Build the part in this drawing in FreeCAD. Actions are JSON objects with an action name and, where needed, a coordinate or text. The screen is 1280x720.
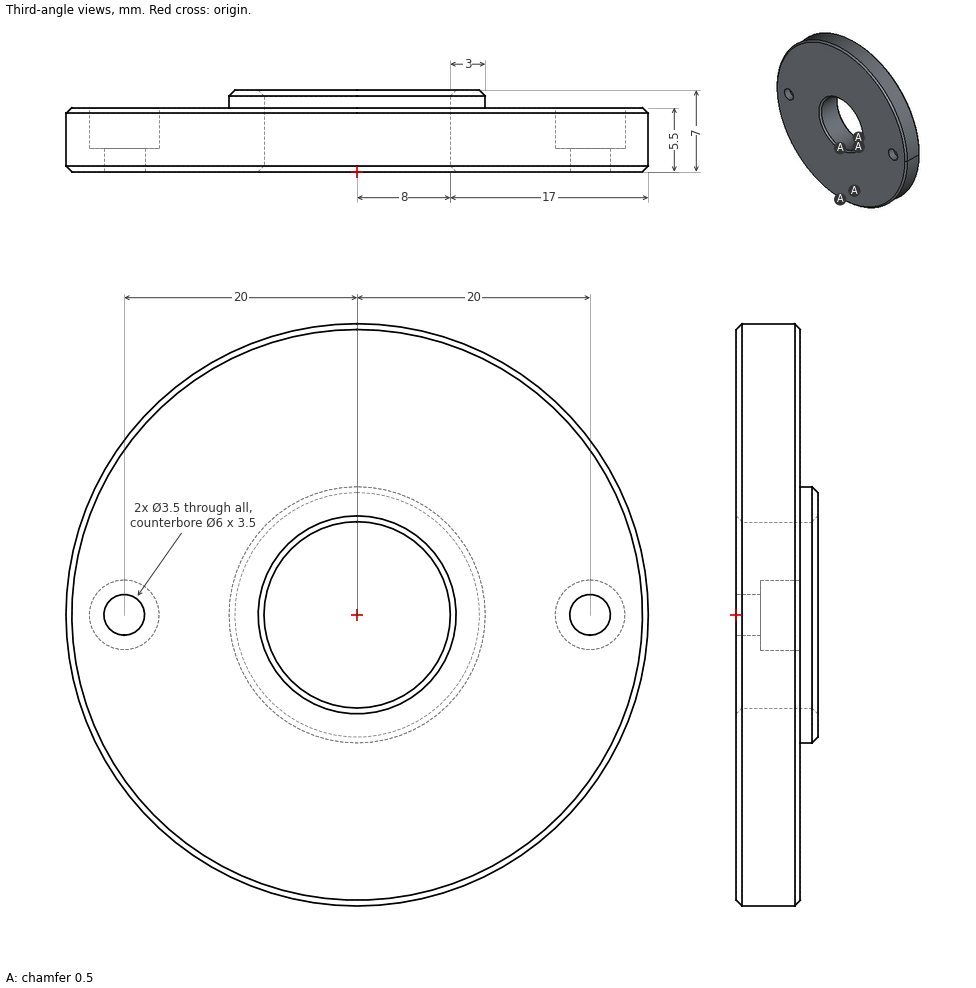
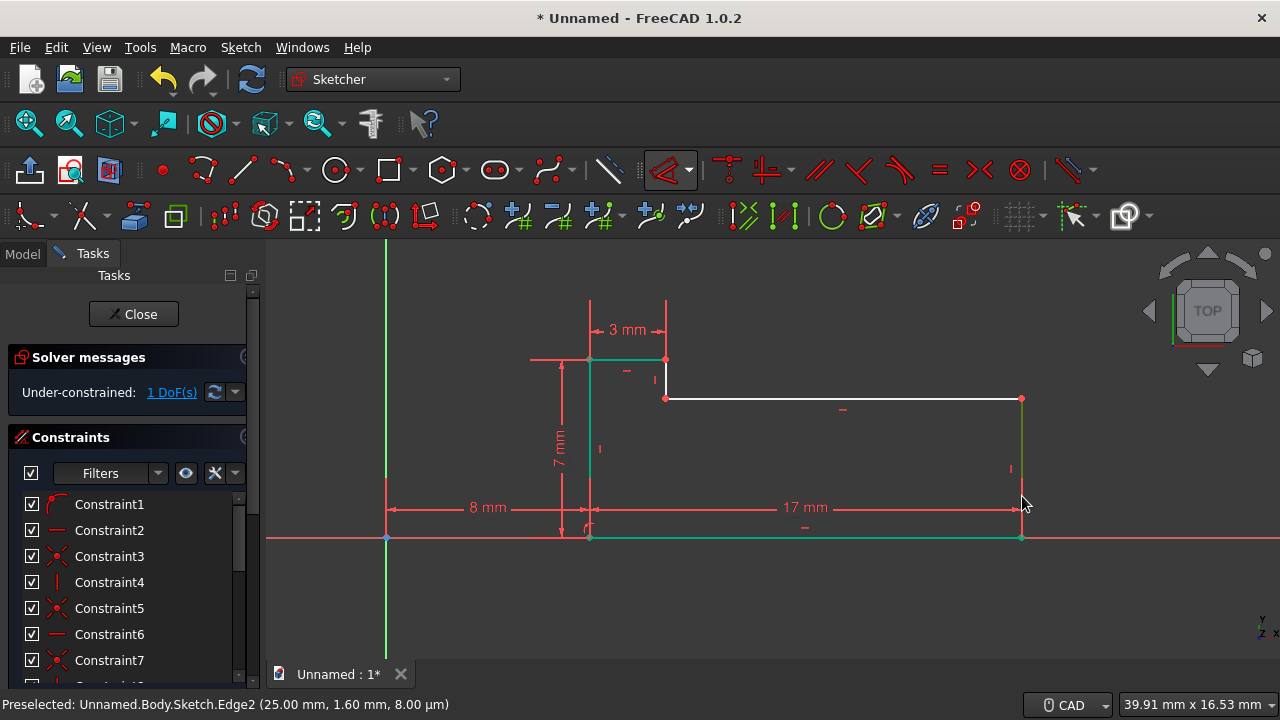
{"action": "left_click", "coordinate": [692, 170]}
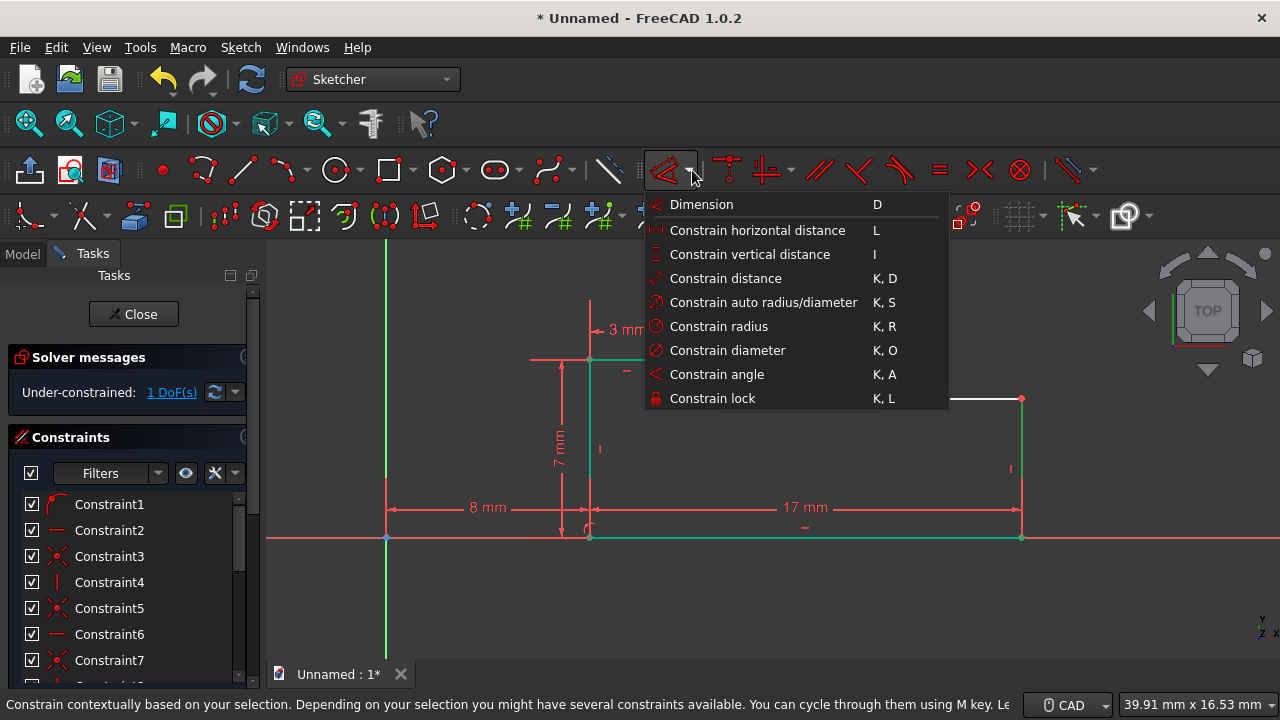
{"action": "left_click", "coordinate": [797, 254]}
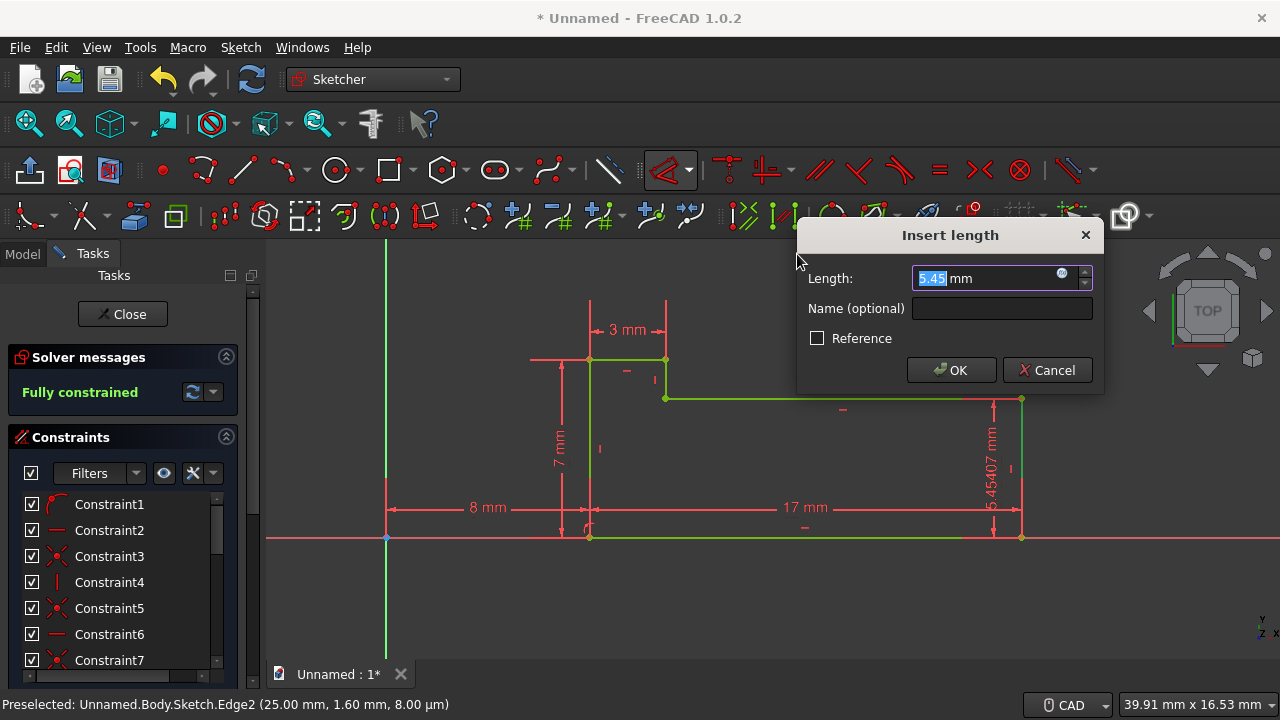
{"action": "type", "text": "5.5"}
{"action": "key", "text": "Return"}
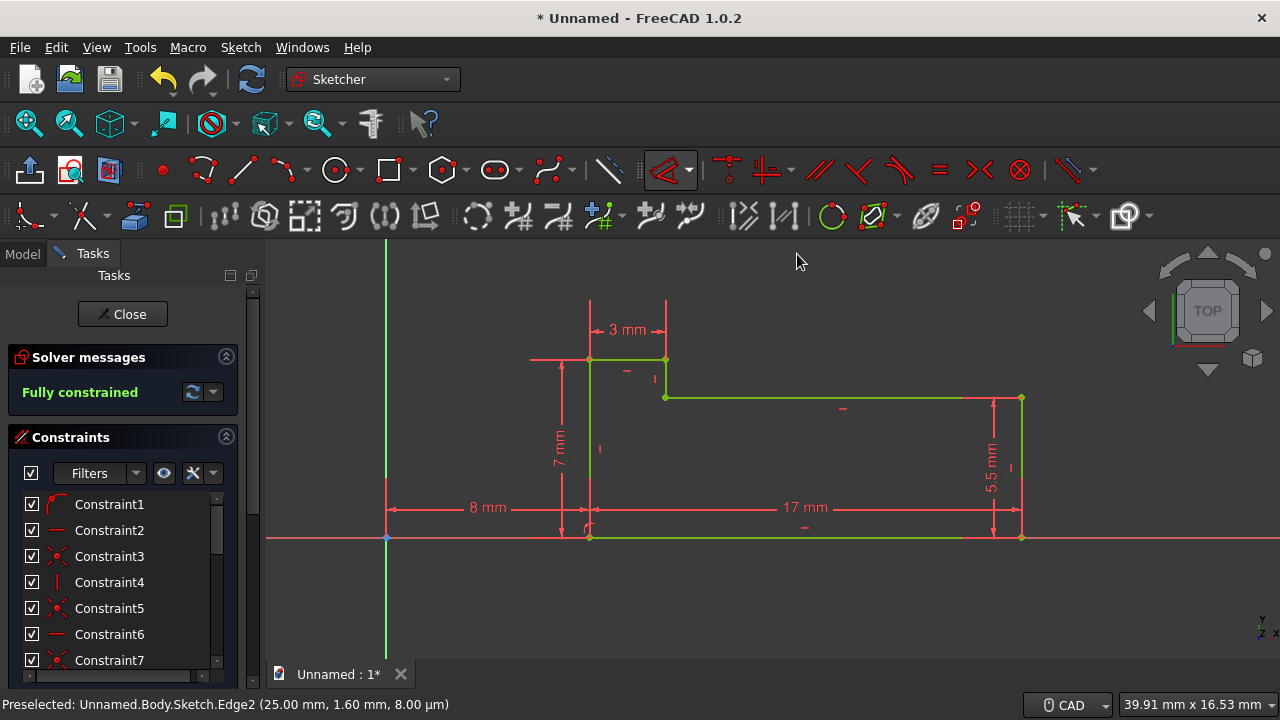
{"action": "left_click", "coordinate": [123, 314]}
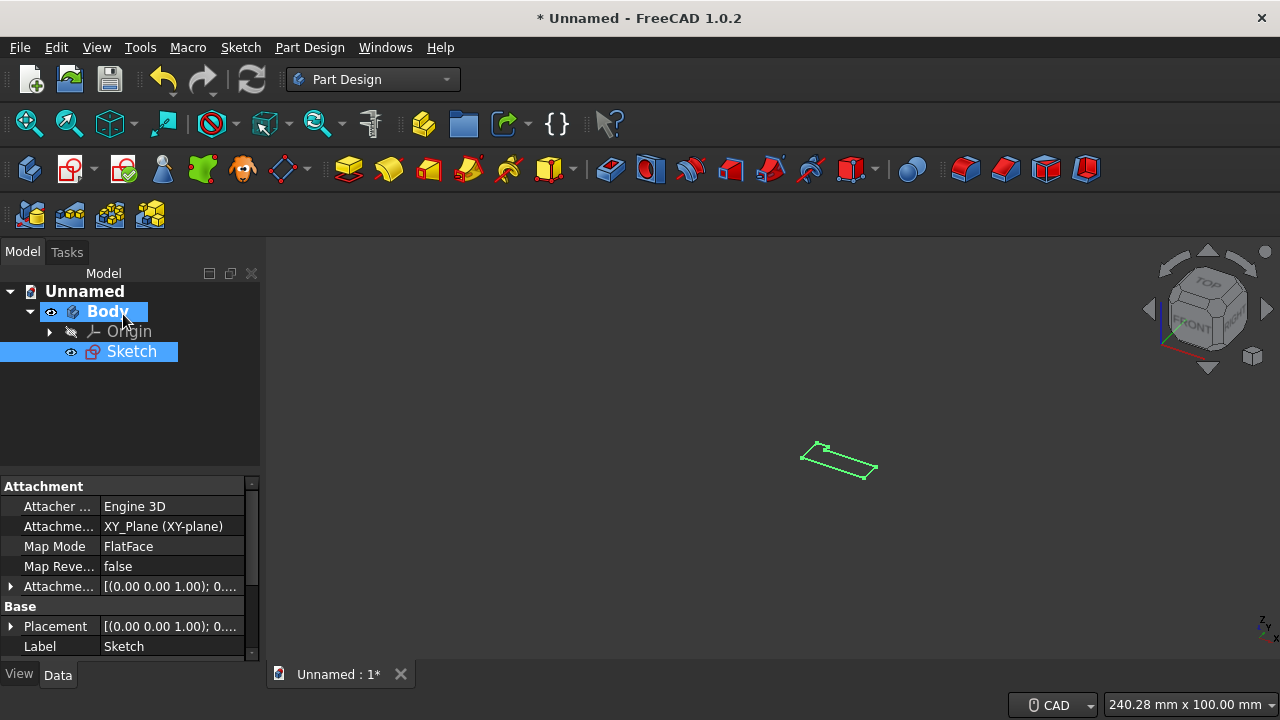
{"action": "left_click", "coordinate": [390, 170]}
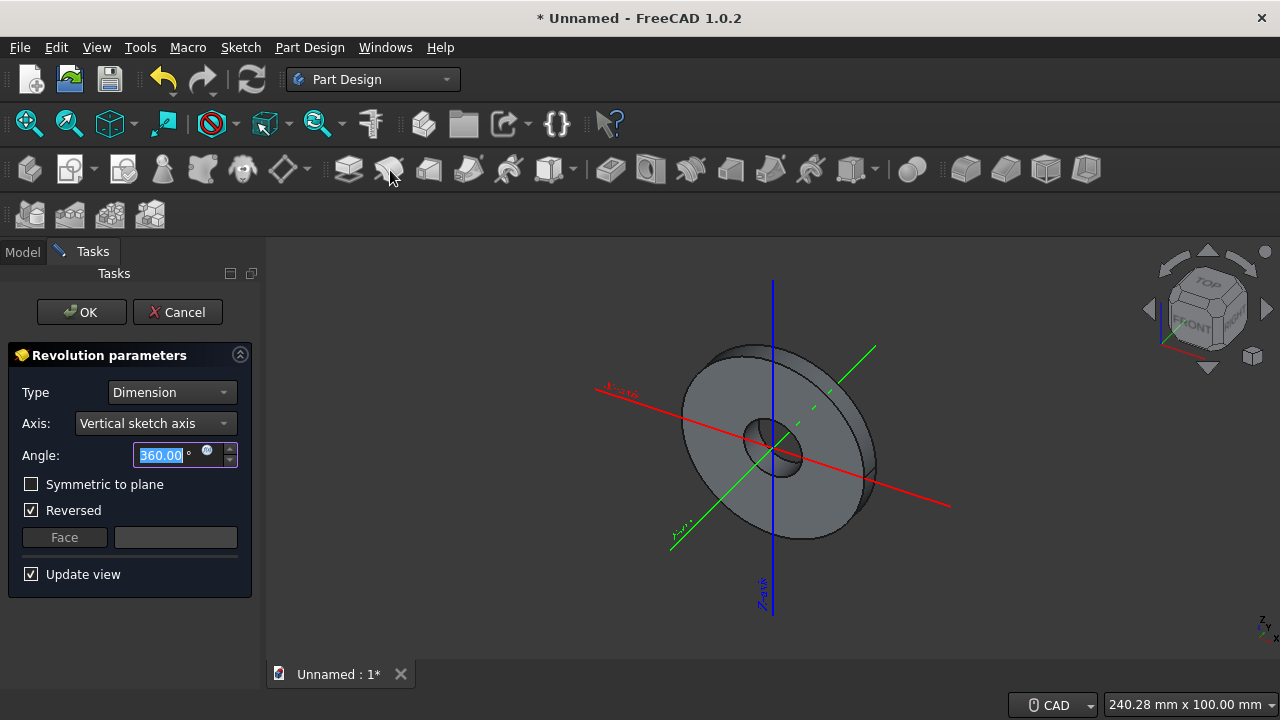
{"action": "left_click", "coordinate": [82, 312]}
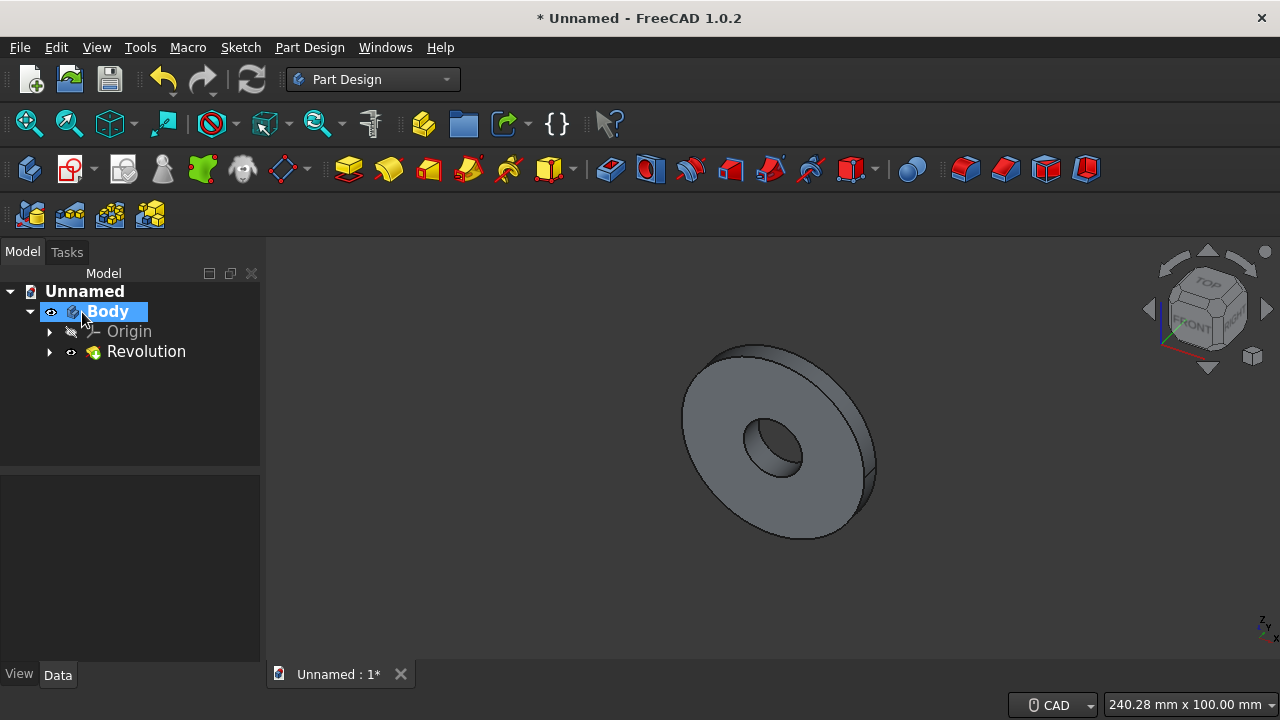
{"action": "key", "text": "4"}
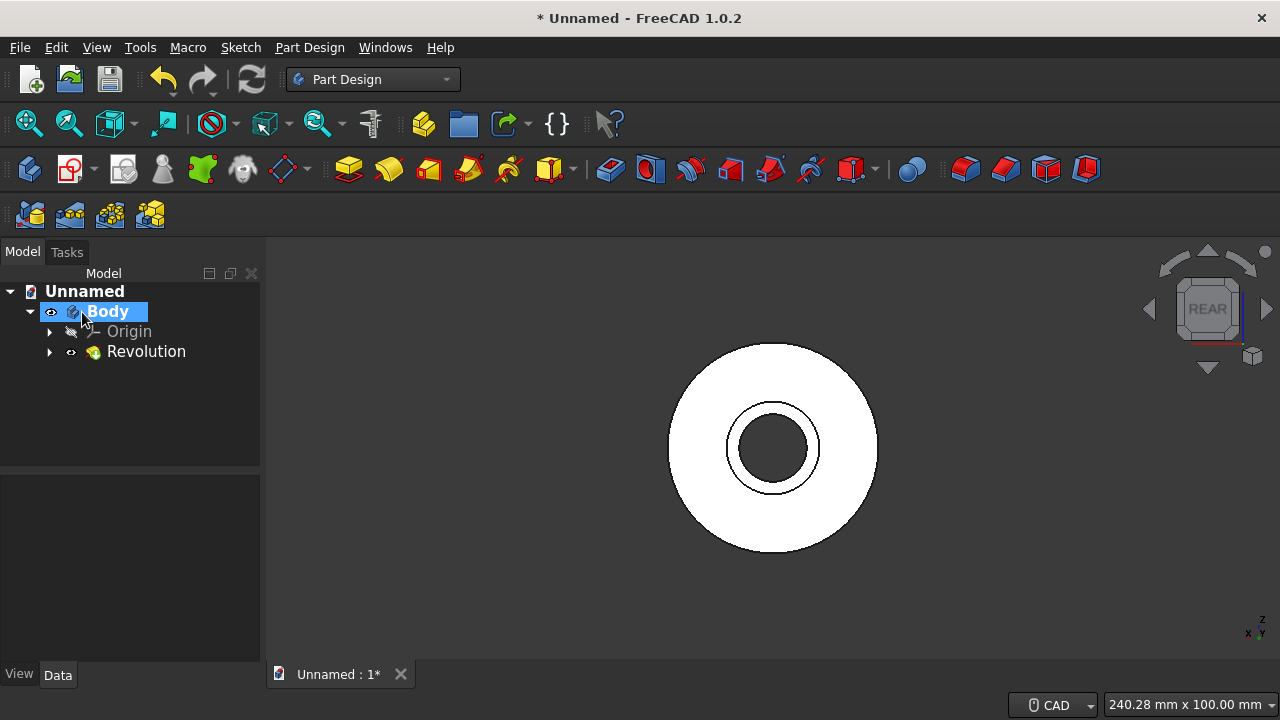
{"action": "left_click", "coordinate": [713, 417]}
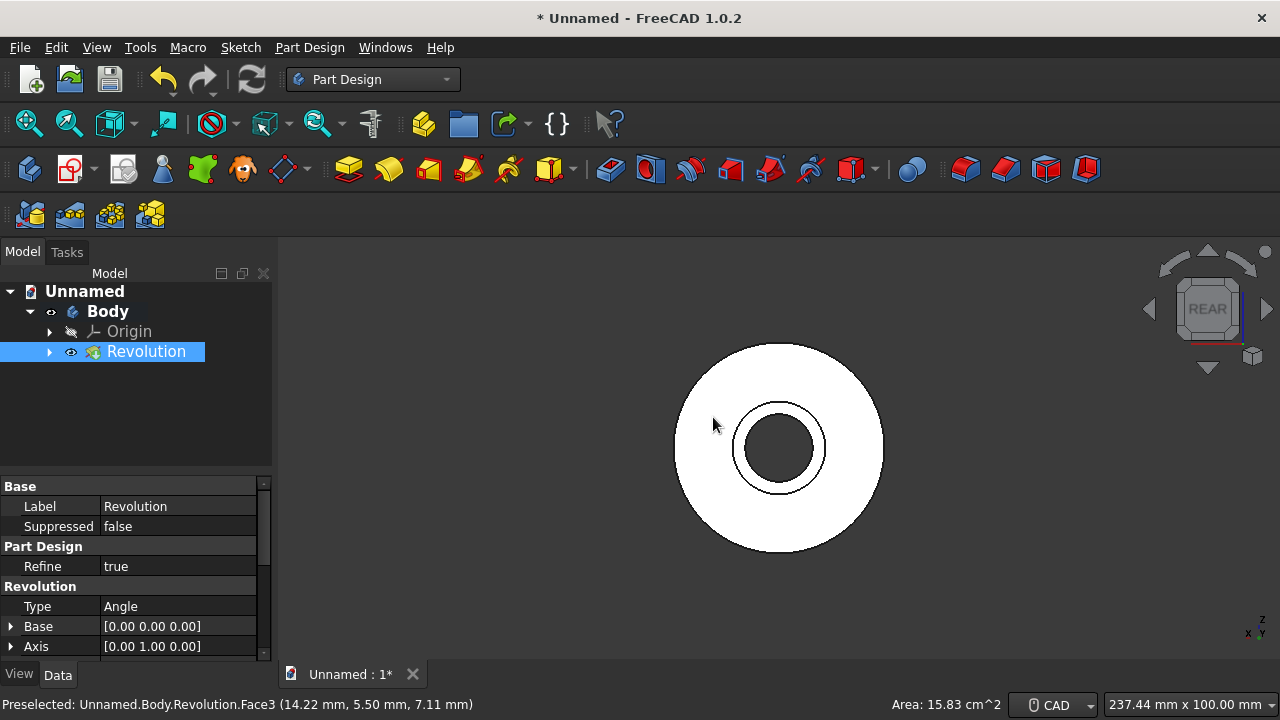
{"action": "left_click", "coordinate": [70, 170]}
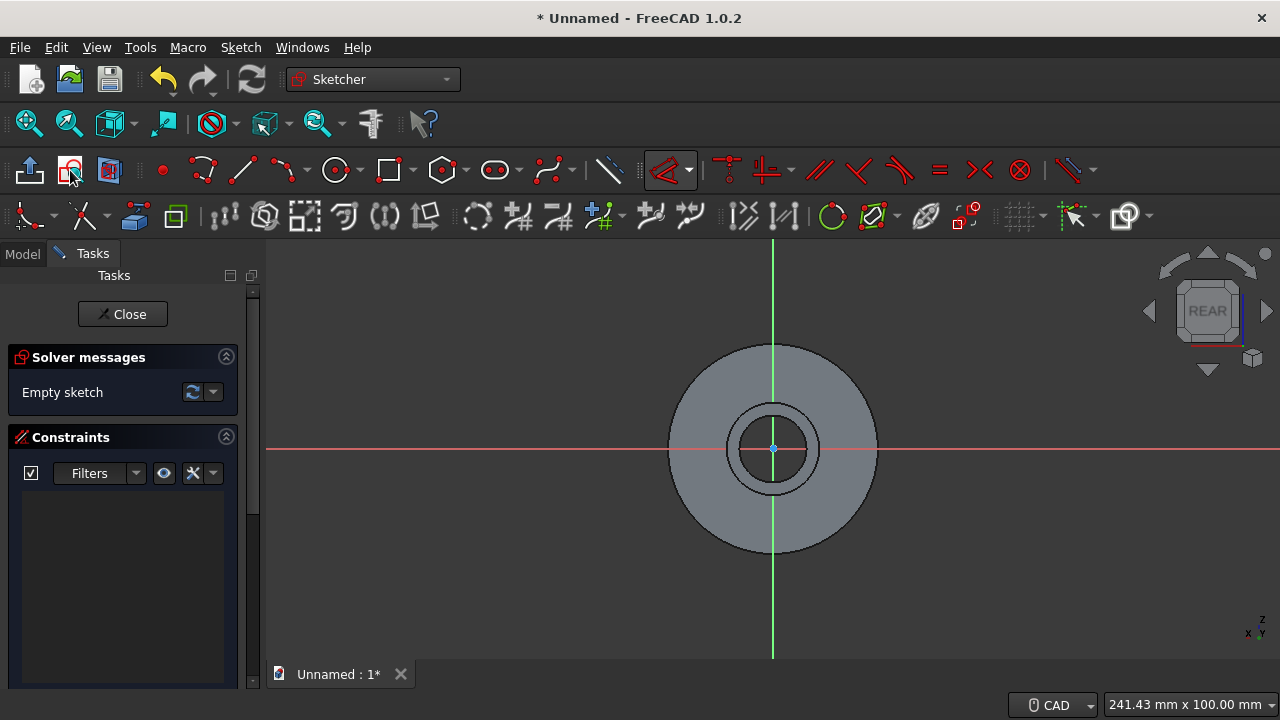
{"action": "scroll", "coordinate": [803, 449], "scroll_direction": "up", "scroll_amount": 6}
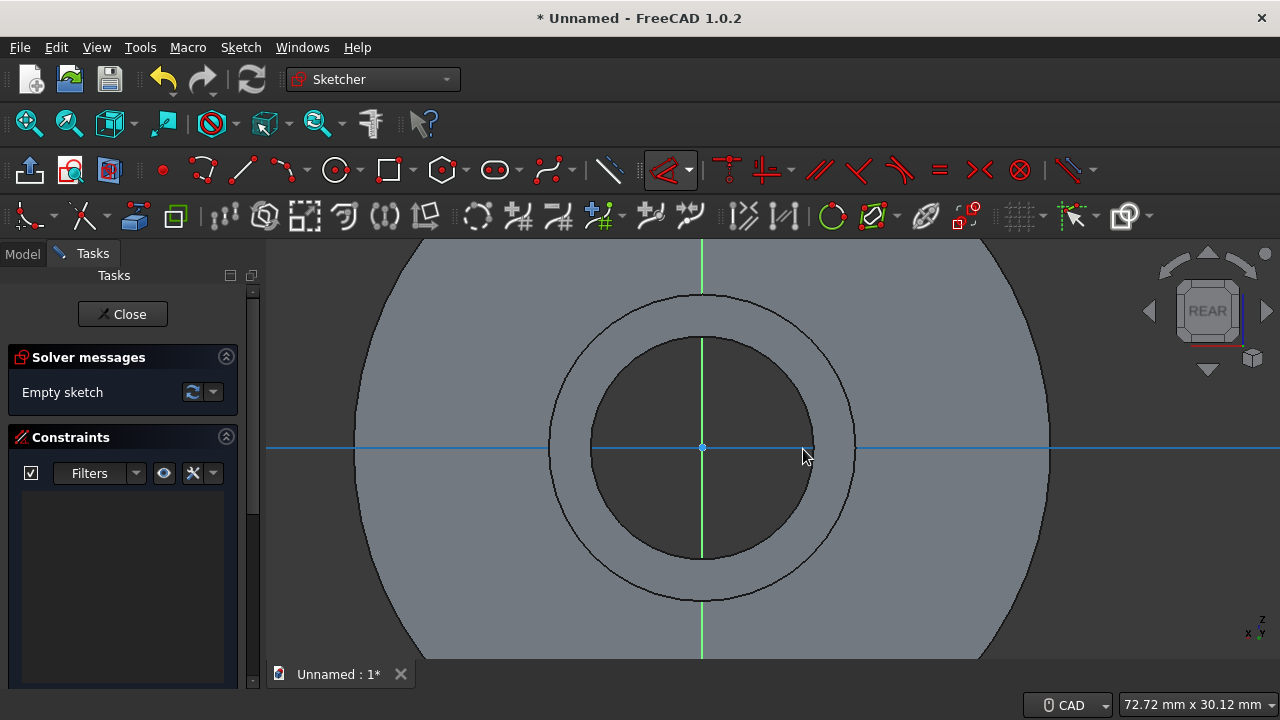
{"action": "left_click", "coordinate": [336, 170]}